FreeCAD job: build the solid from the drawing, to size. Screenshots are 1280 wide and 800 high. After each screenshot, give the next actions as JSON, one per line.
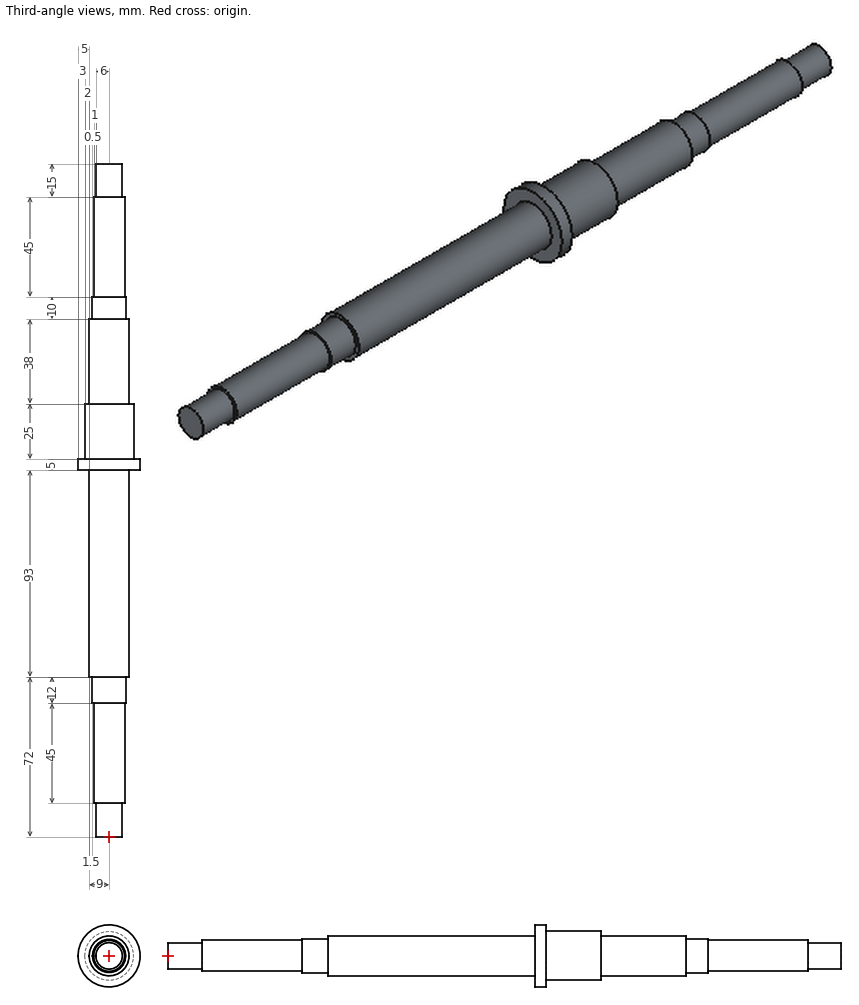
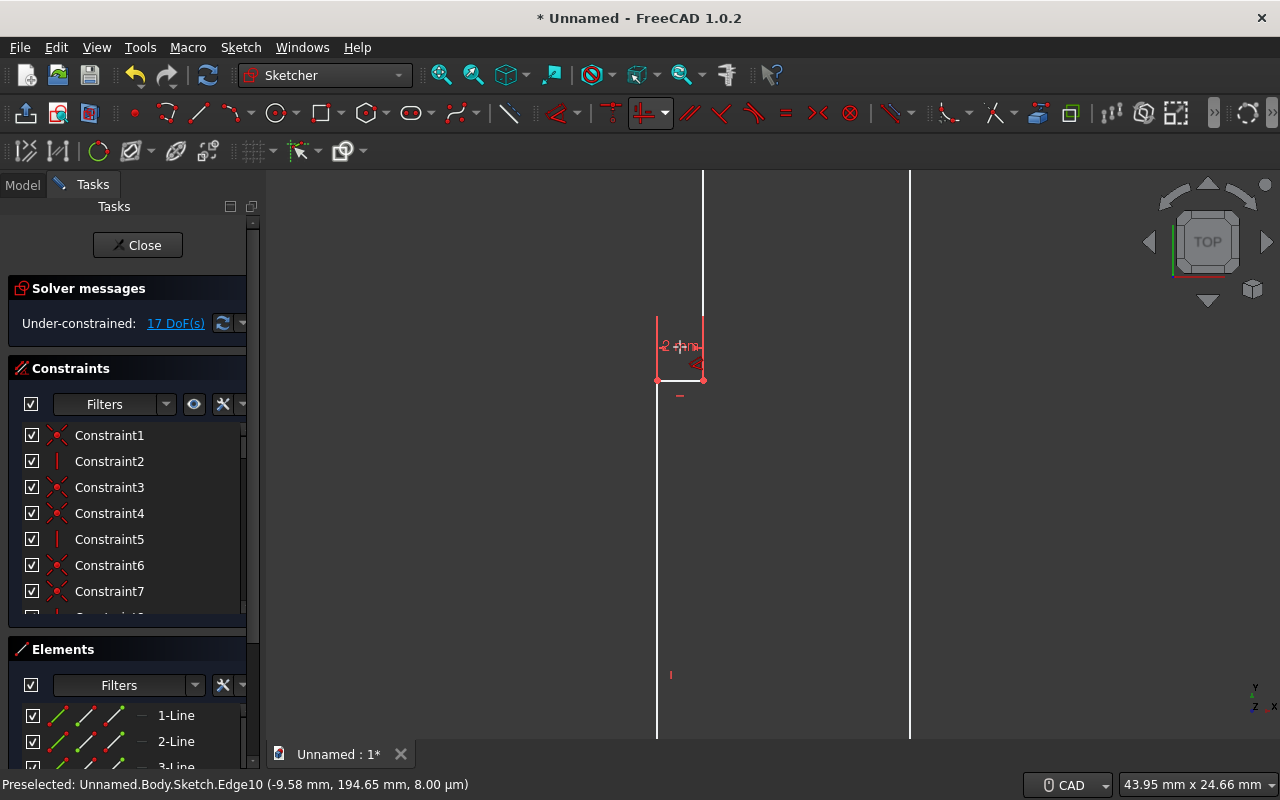
{"action": "scroll", "coordinate": [702, 406], "scroll_direction": "down", "scroll_amount": 15}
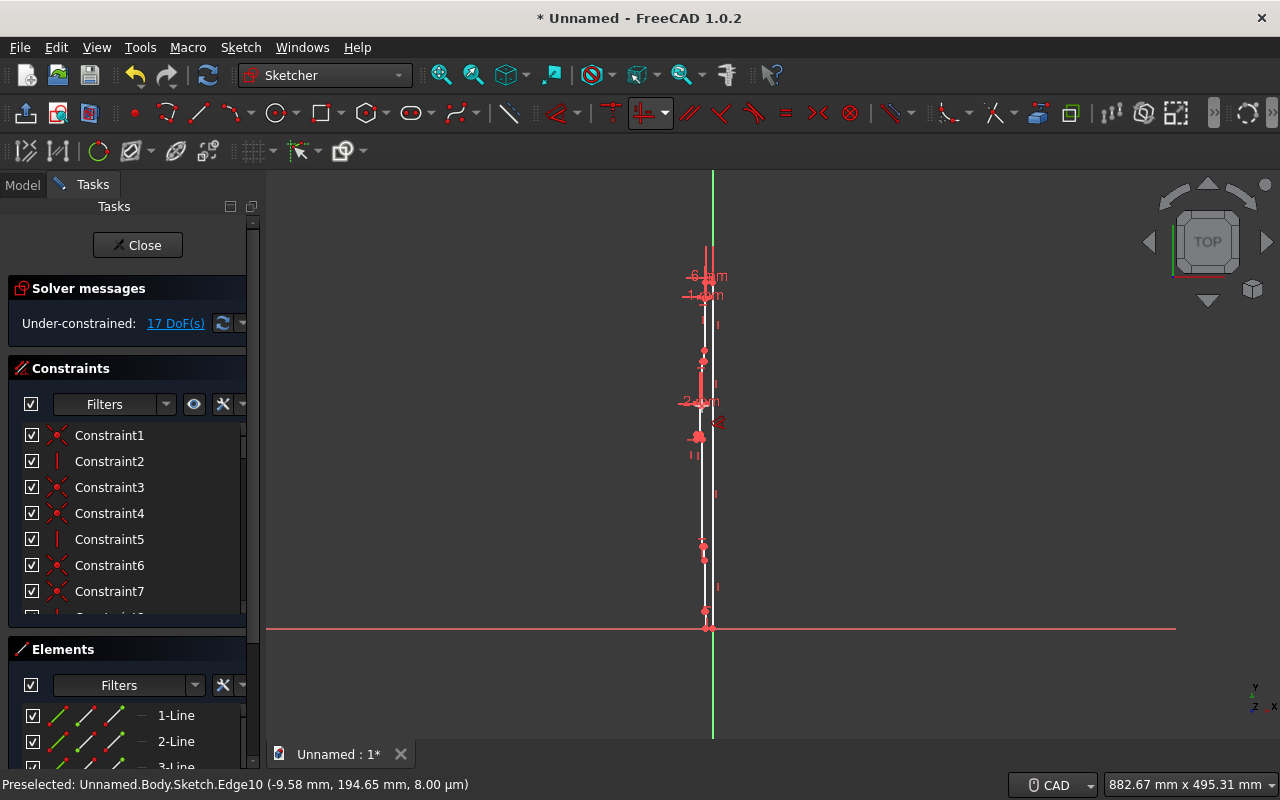
{"action": "scroll", "coordinate": [699, 434], "scroll_direction": "up", "scroll_amount": 13}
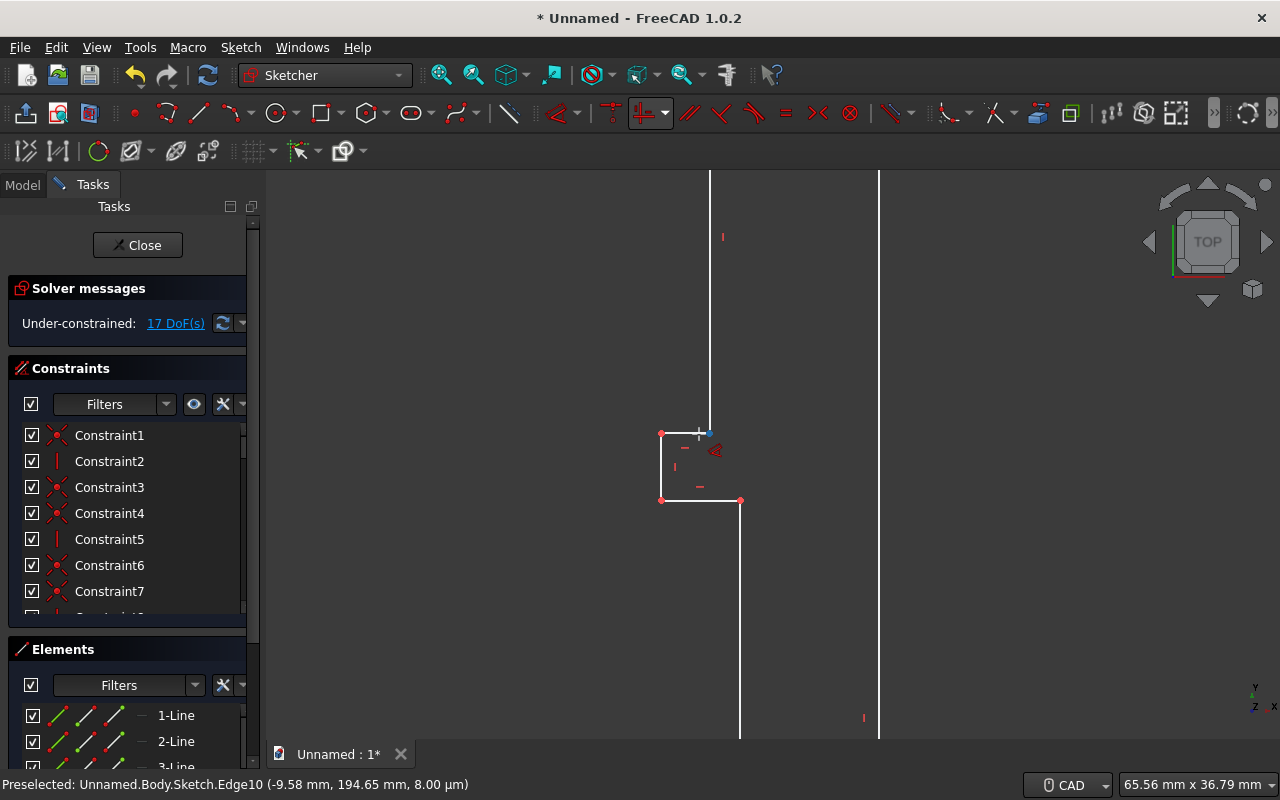
{"action": "left_click", "coordinate": [695, 433]}
{"action": "left_click", "coordinate": [685, 399]}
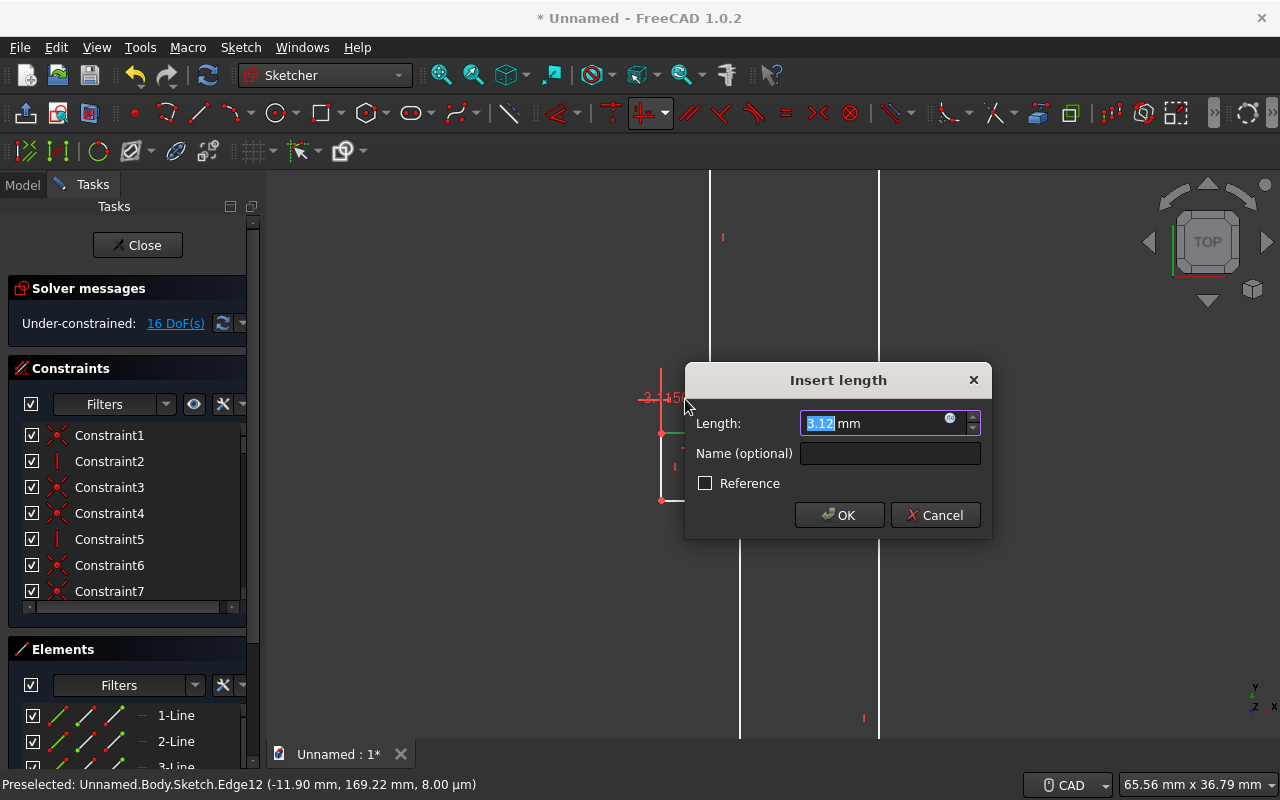
{"action": "type", "text": "3"}
{"action": "key", "text": "Return"}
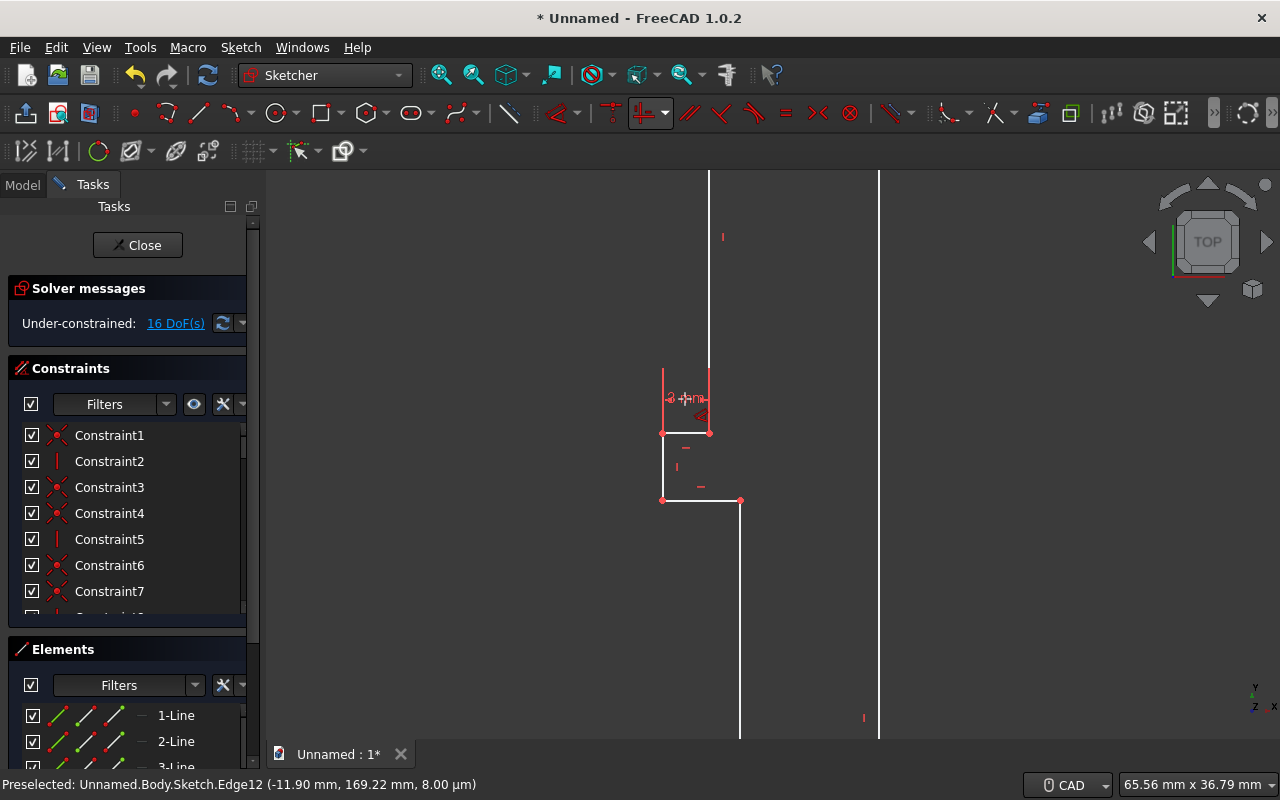
{"action": "left_click", "coordinate": [663, 453]}
{"action": "left_click", "coordinate": [629, 467]}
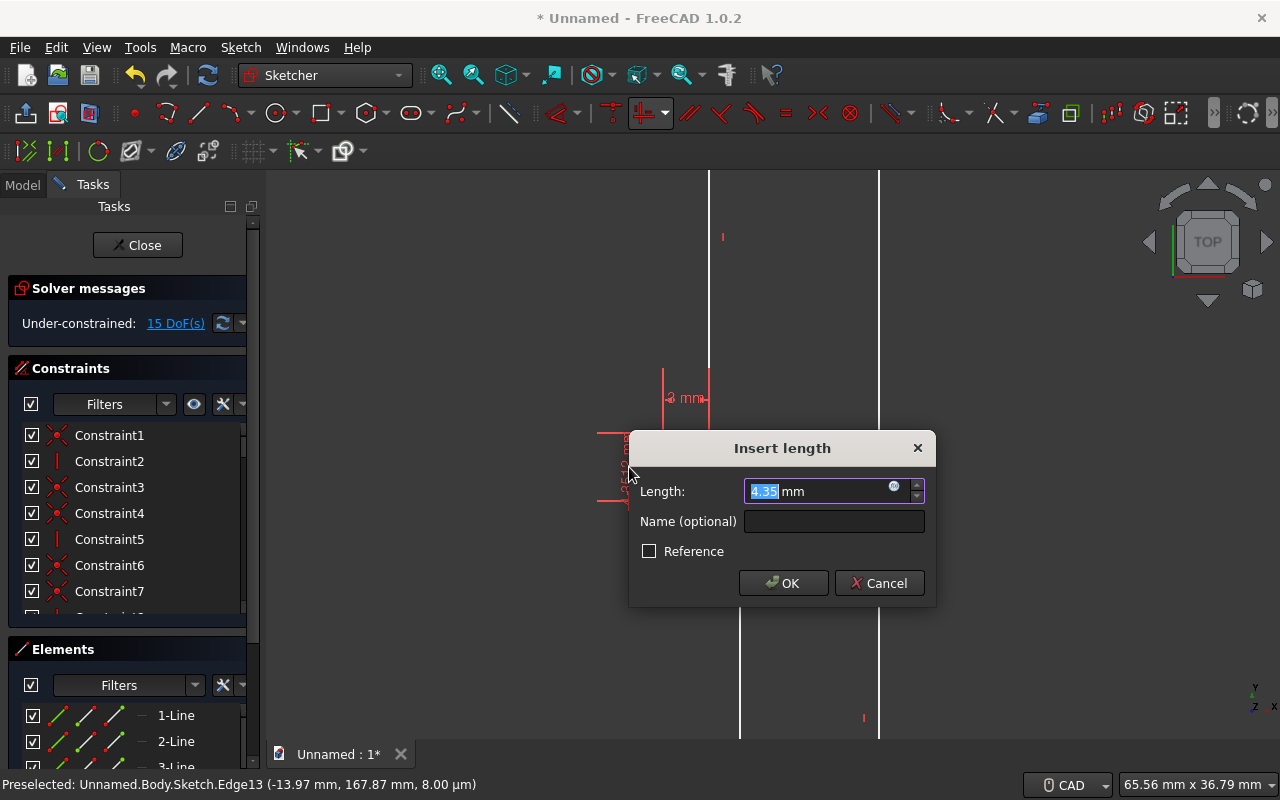
{"action": "type", "text": "5"}
{"action": "key", "text": "Return"}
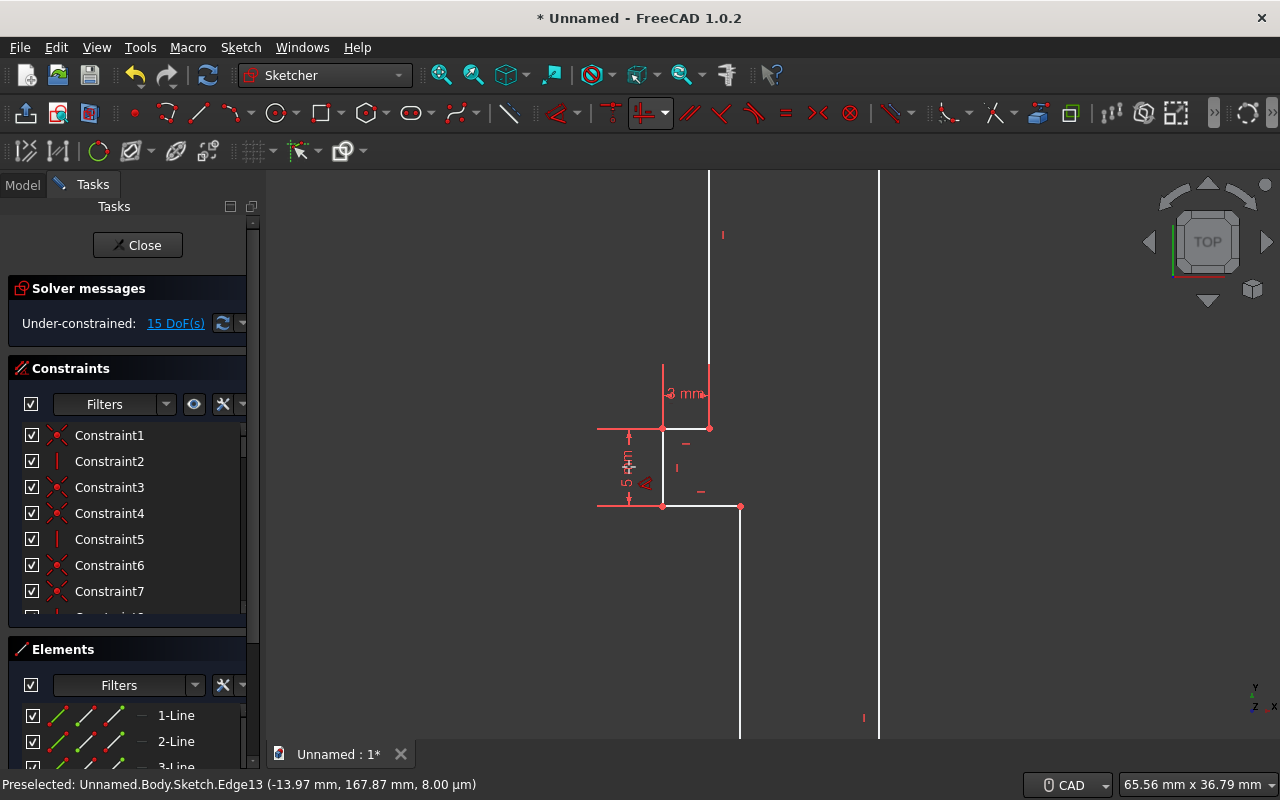
{"action": "left_click", "coordinate": [686, 506]}
{"action": "left_click", "coordinate": [702, 472]}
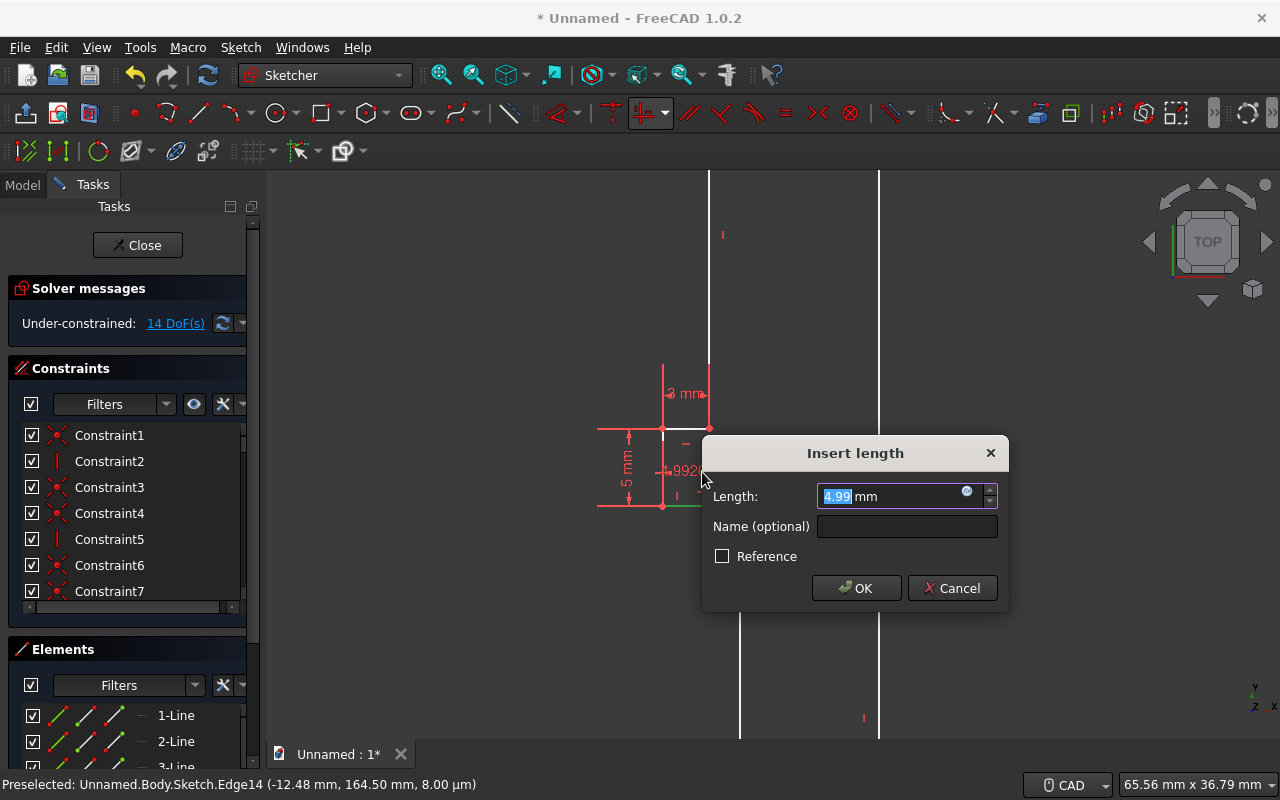
{"action": "type", "text": "5"}
{"action": "key", "text": "Return"}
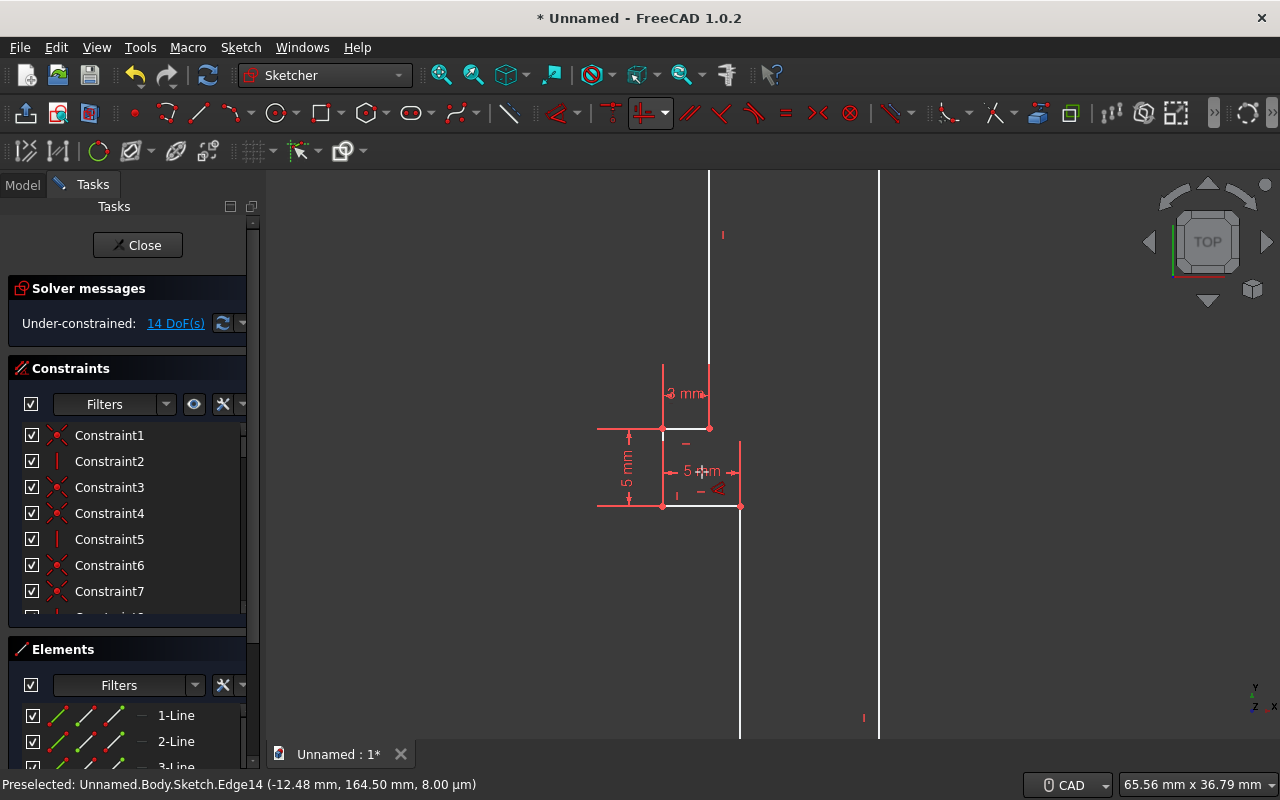
{"action": "scroll", "coordinate": [699, 434], "scroll_direction": "down", "scroll_amount": 13}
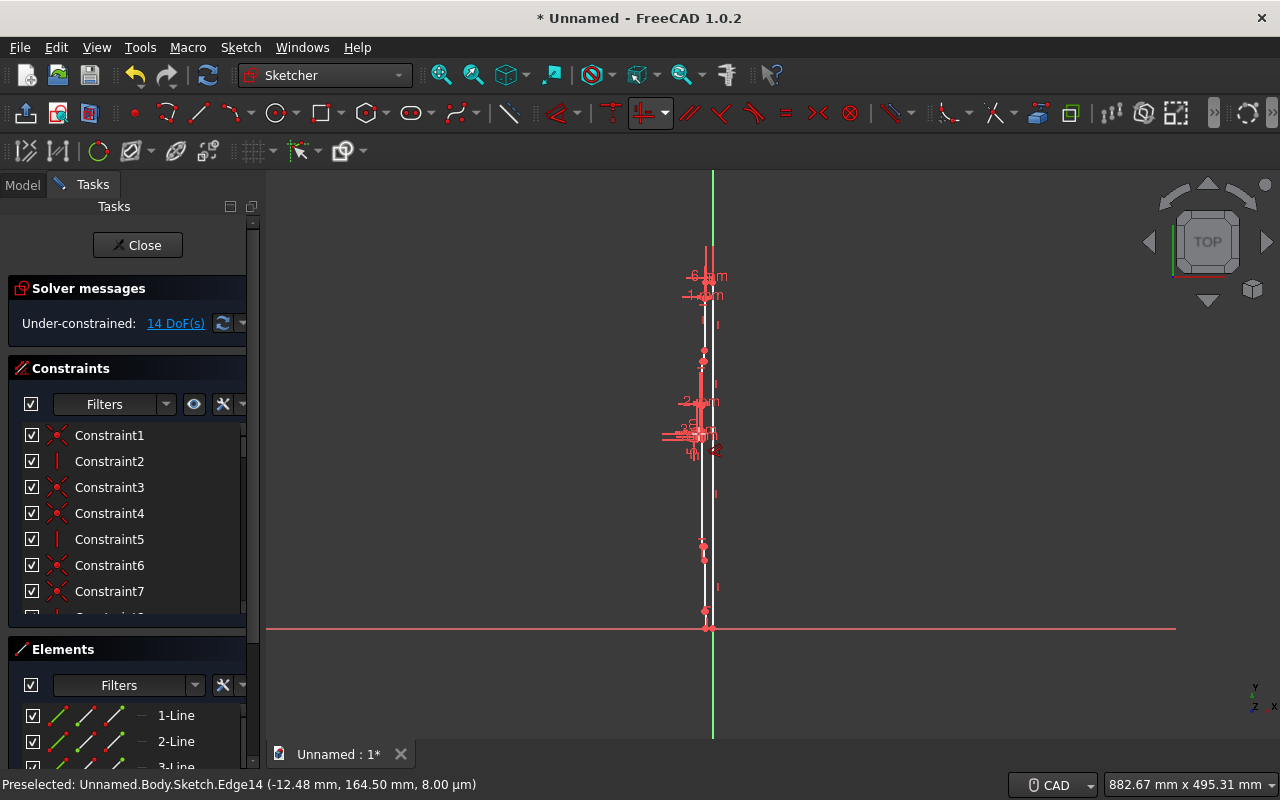
{"action": "scroll", "coordinate": [705, 612], "scroll_direction": "up", "scroll_amount": 18}